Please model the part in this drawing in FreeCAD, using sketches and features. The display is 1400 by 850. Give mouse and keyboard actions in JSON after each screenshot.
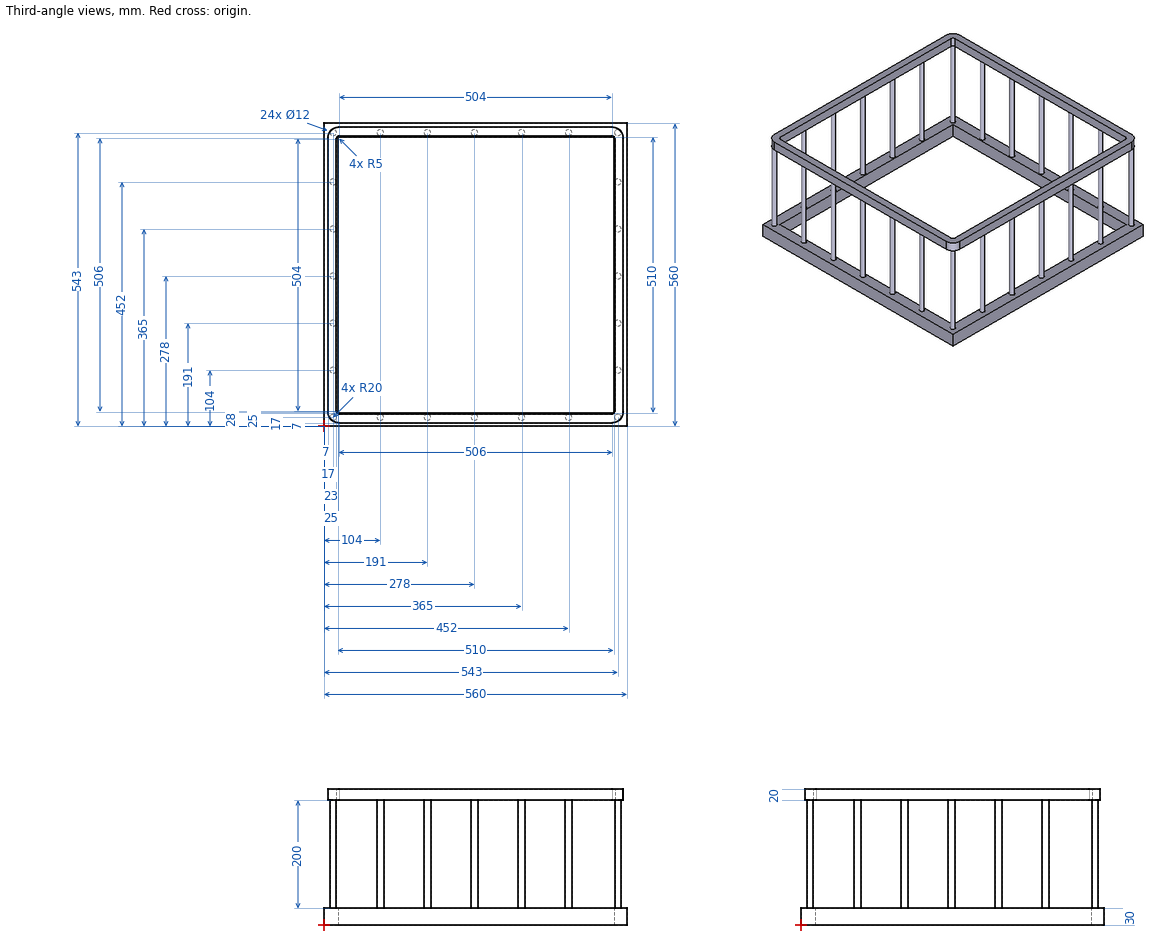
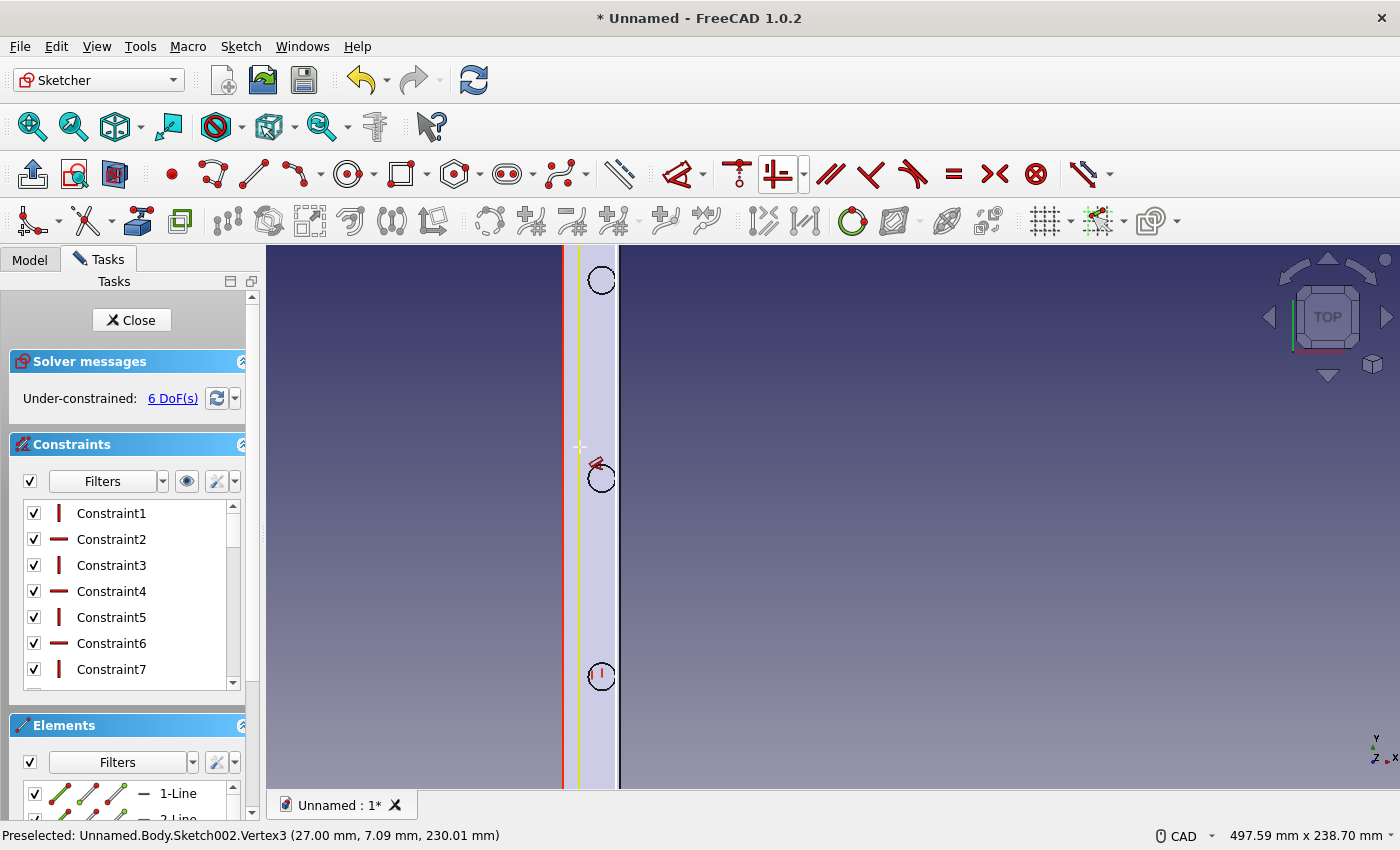
{"action": "left_click", "coordinate": [579, 445]}
{"action": "left_click", "coordinate": [545, 517]}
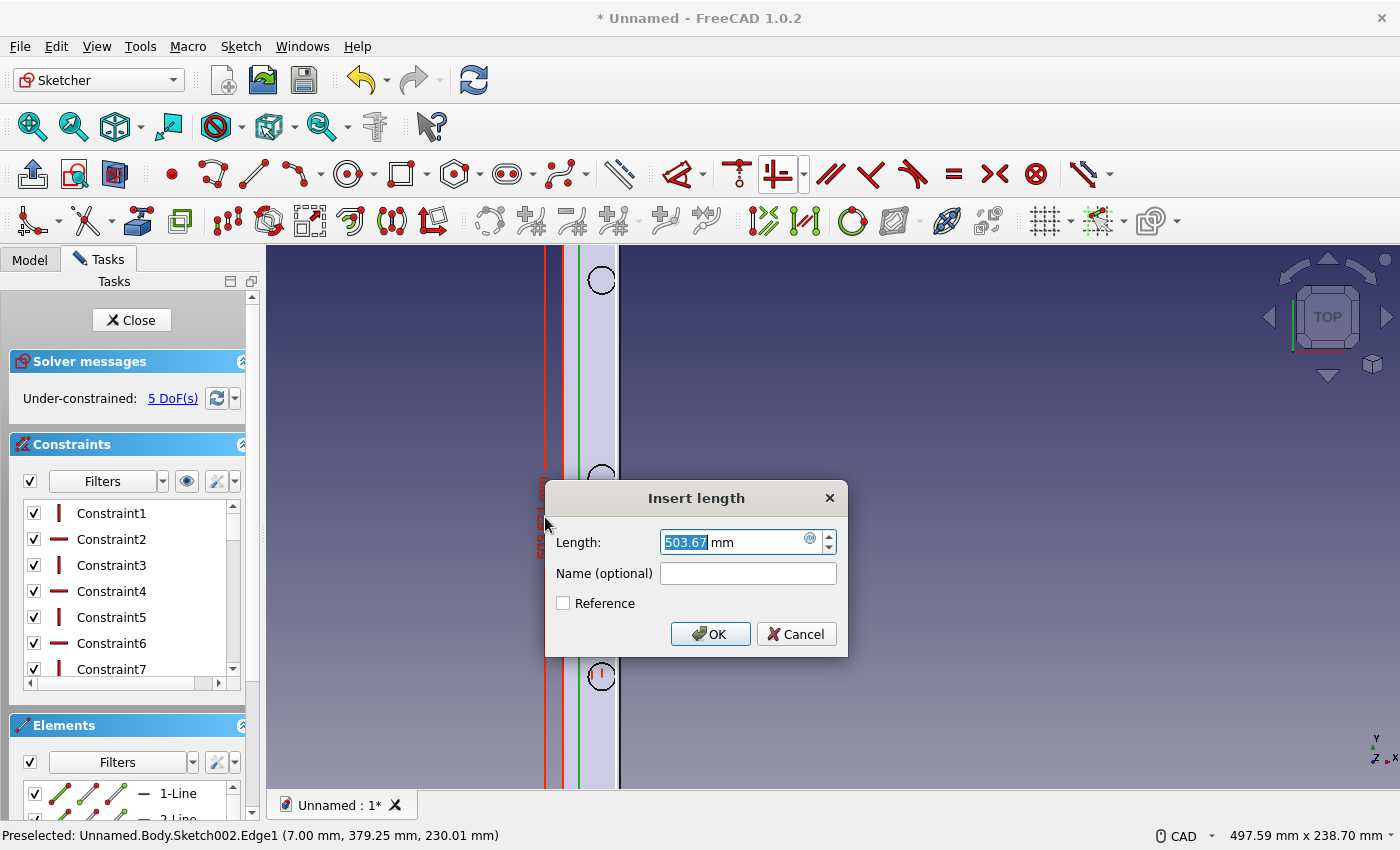
{"action": "type", "text": "506"}
{"action": "key", "text": "Return"}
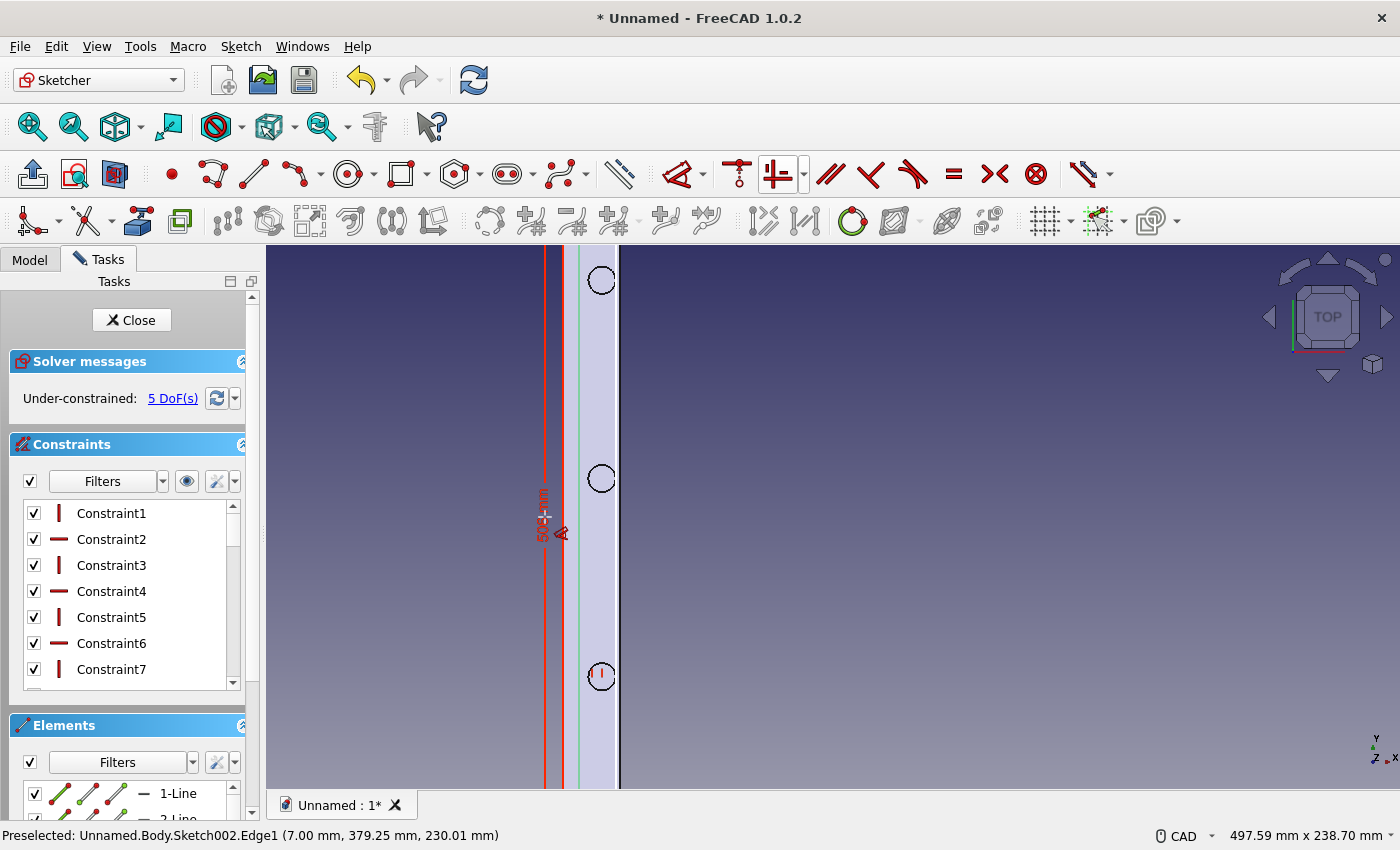
{"action": "scroll", "coordinate": [580, 447], "scroll_direction": "down", "scroll_amount": 6}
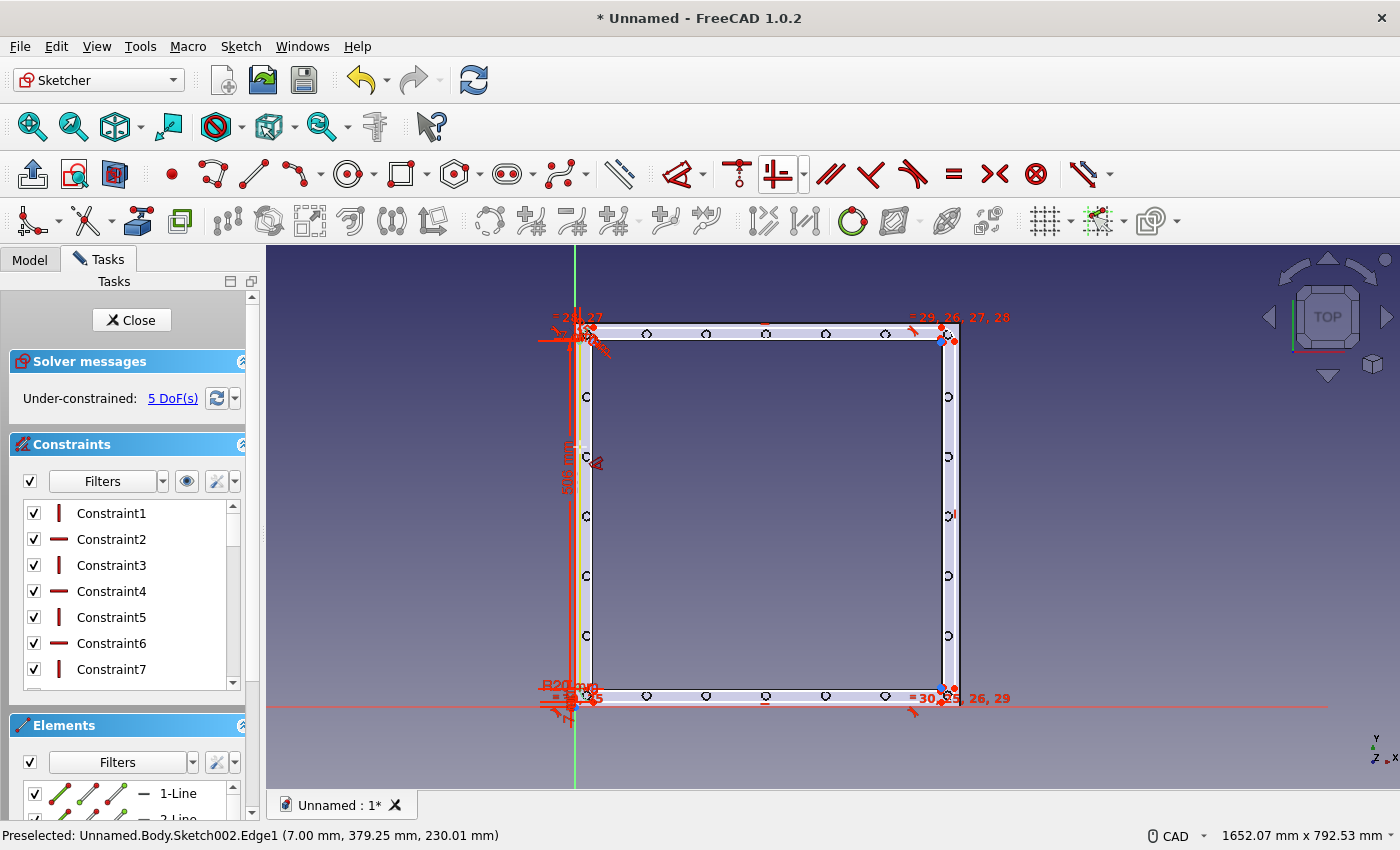
{"action": "scroll", "coordinate": [698, 702], "scroll_direction": "up", "scroll_amount": 6}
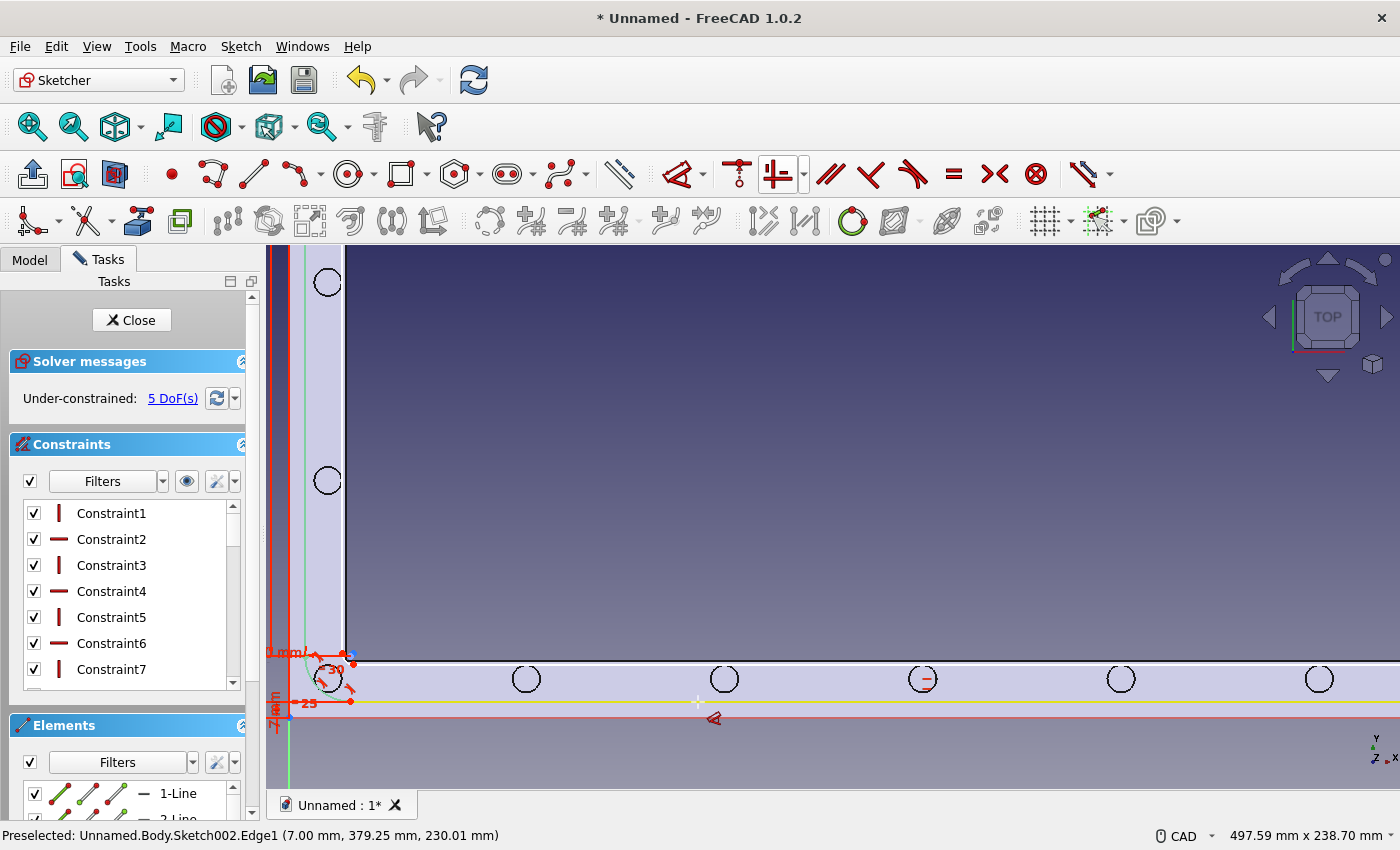
{"action": "left_click", "coordinate": [697, 702]}
{"action": "left_click", "coordinate": [793, 736]}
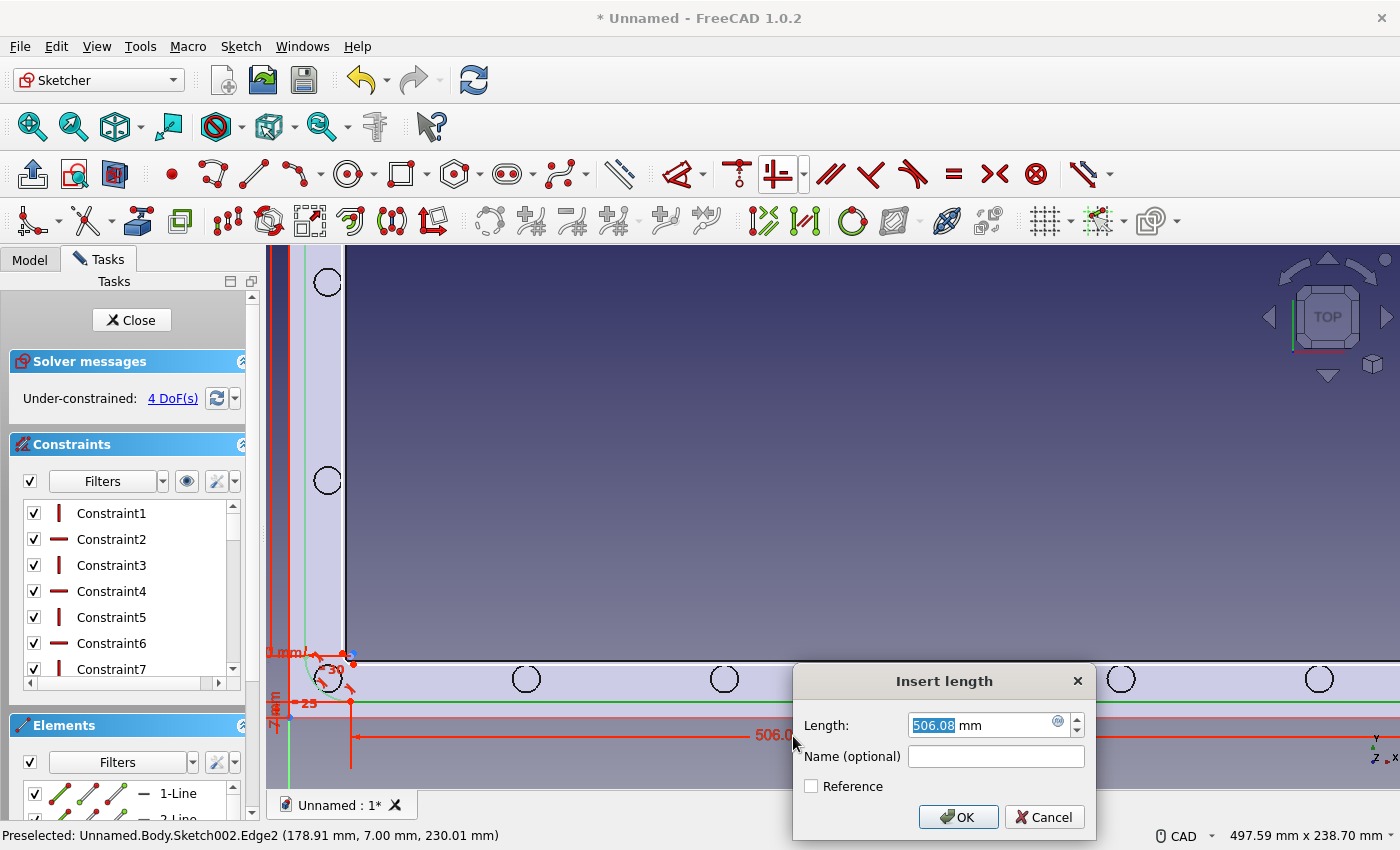
{"action": "type", "text": "506"}
{"action": "key", "text": "Return"}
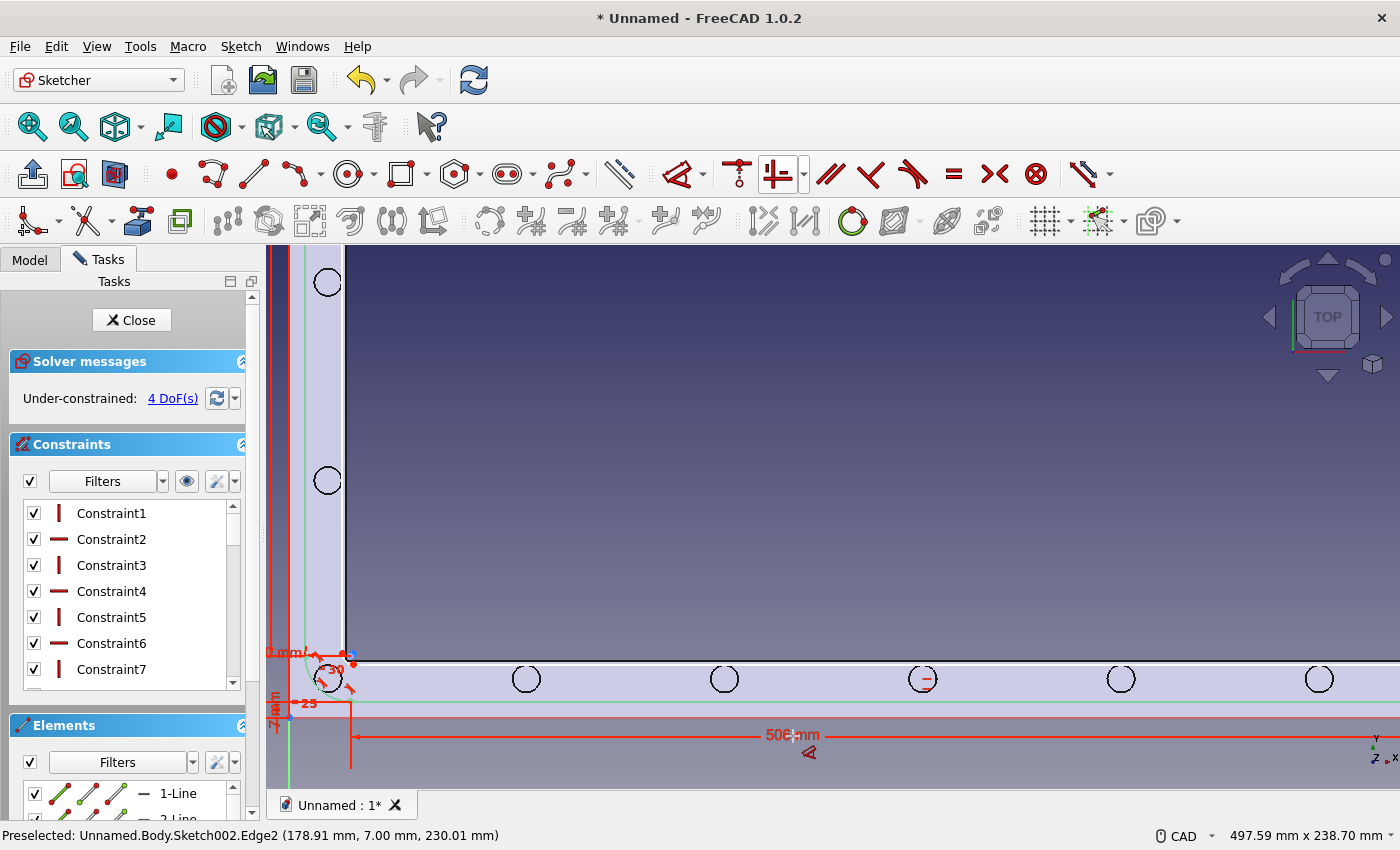
{"action": "left_click", "coordinate": [342, 309]}
{"action": "left_click", "coordinate": [376, 463]}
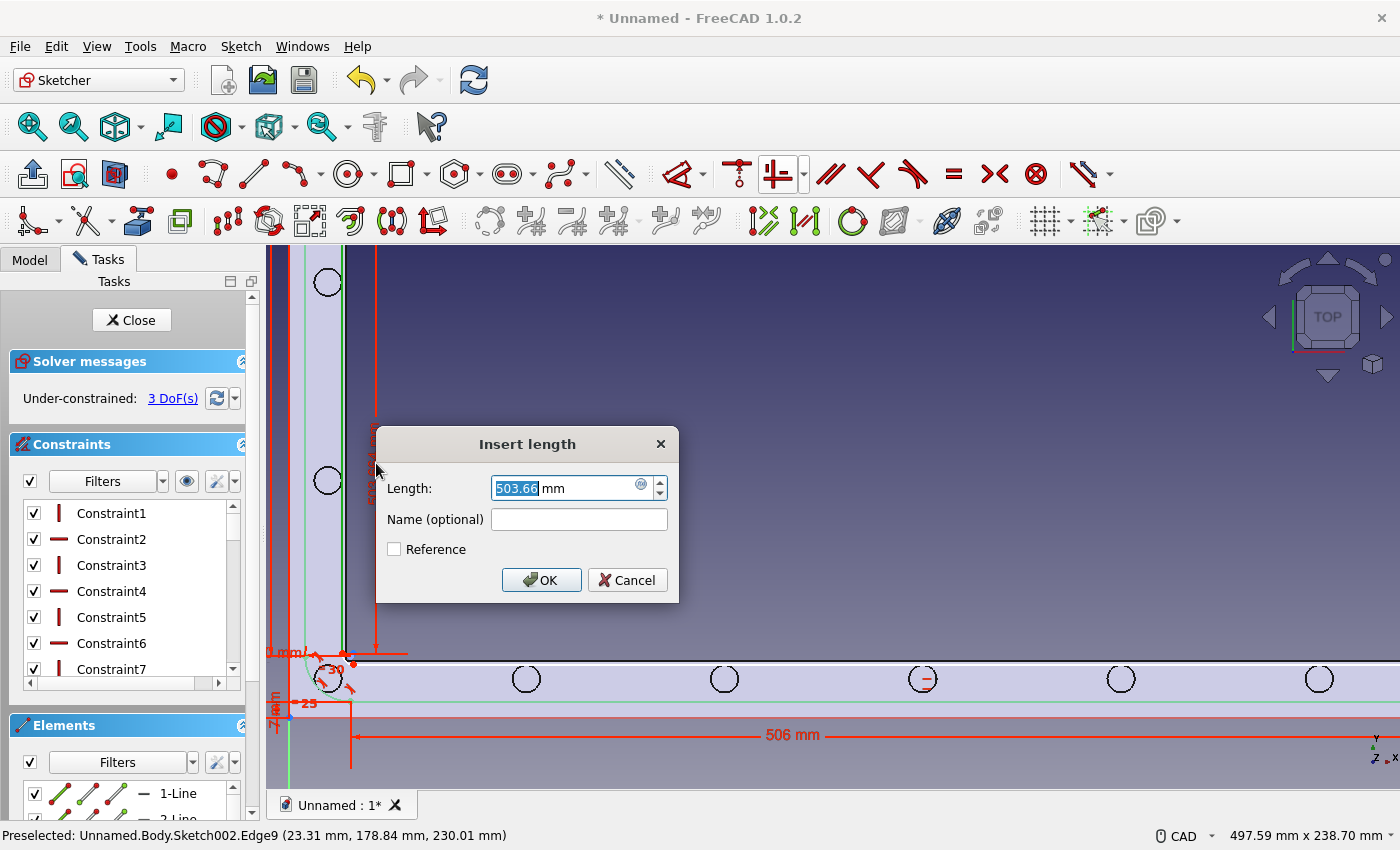
{"action": "type", "text": "504"}
{"action": "key", "text": "Return"}